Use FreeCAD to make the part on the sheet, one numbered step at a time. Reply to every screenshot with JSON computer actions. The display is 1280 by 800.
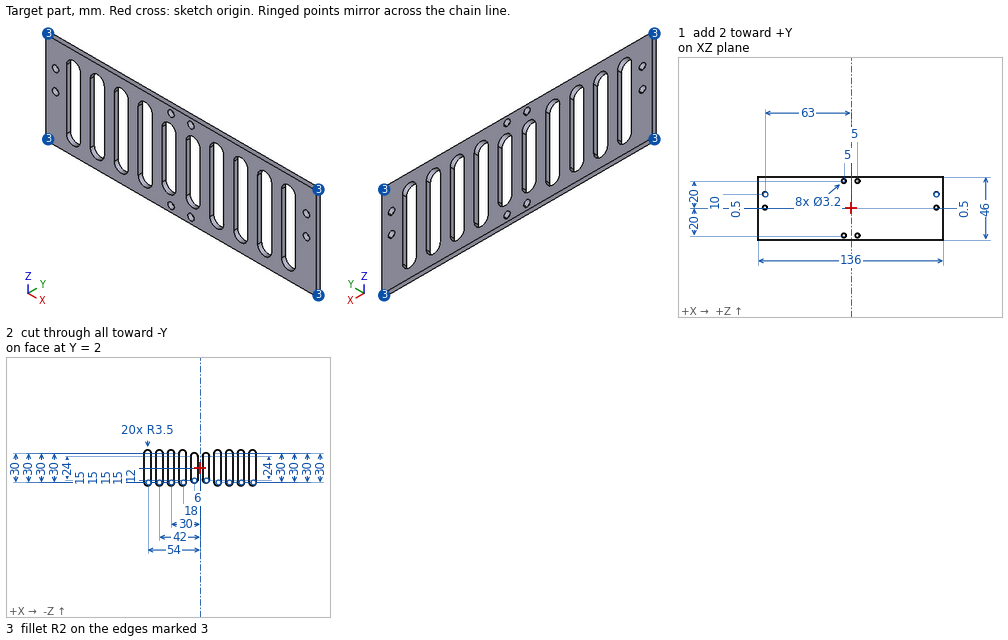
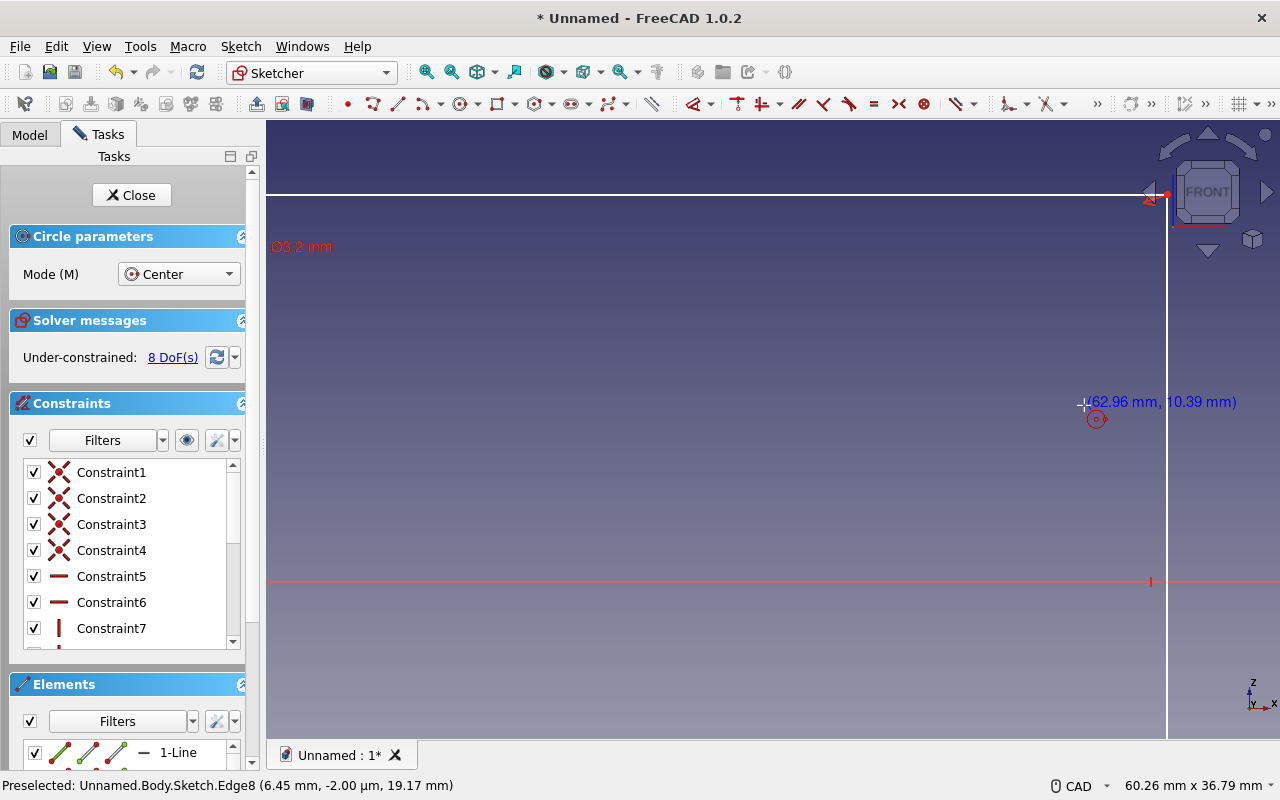
{"action": "scroll", "coordinate": [927, 380], "scroll_direction": "down", "scroll_amount": 7}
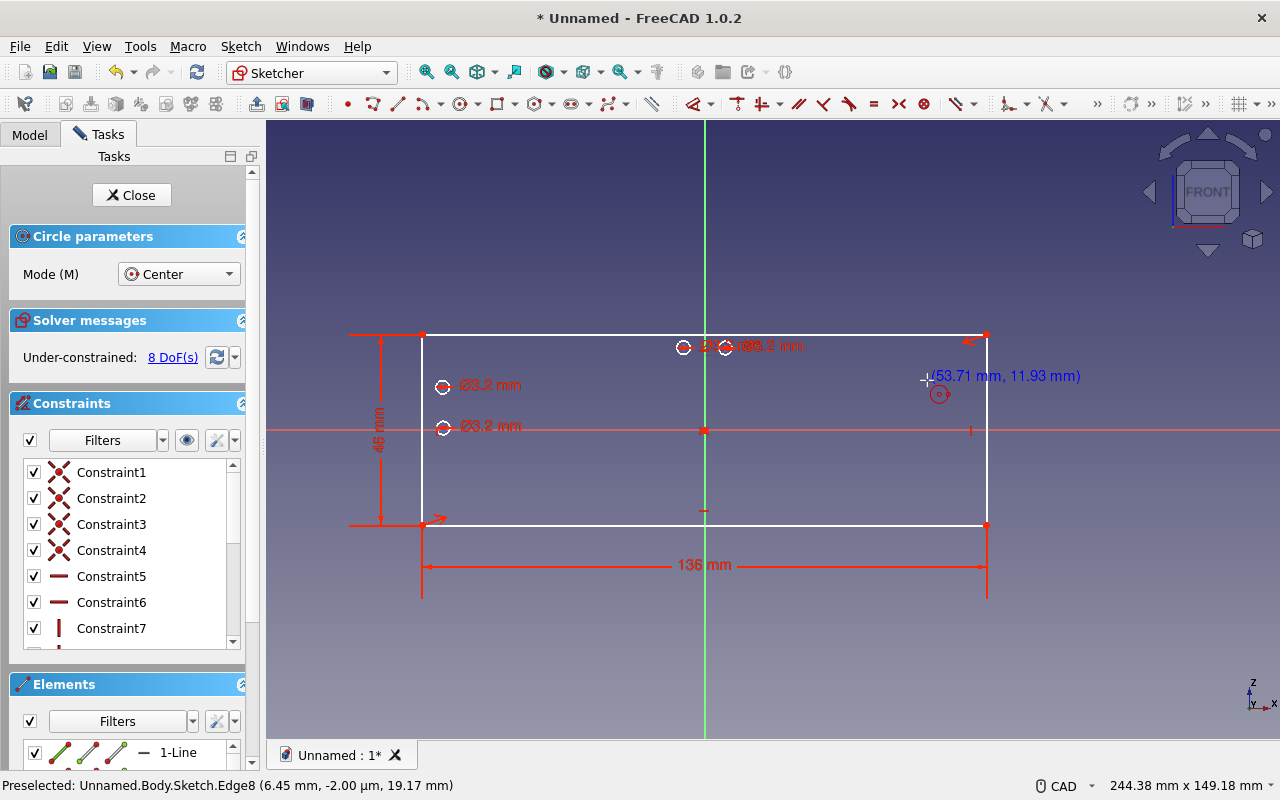
{"action": "left_click", "coordinate": [966, 387]}
{"action": "mouse_move", "coordinate": [971, 382]}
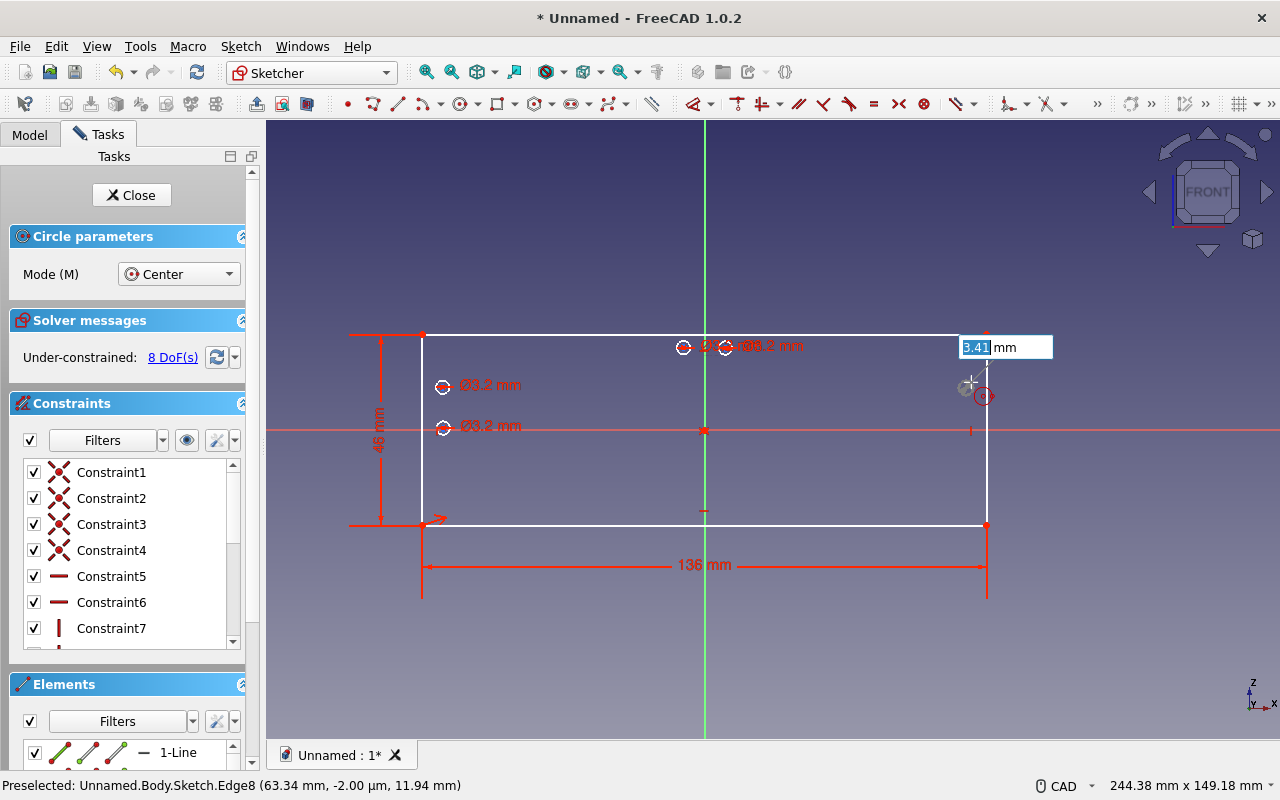
{"action": "type", "text": "3.2"}
{"action": "key", "text": "Return"}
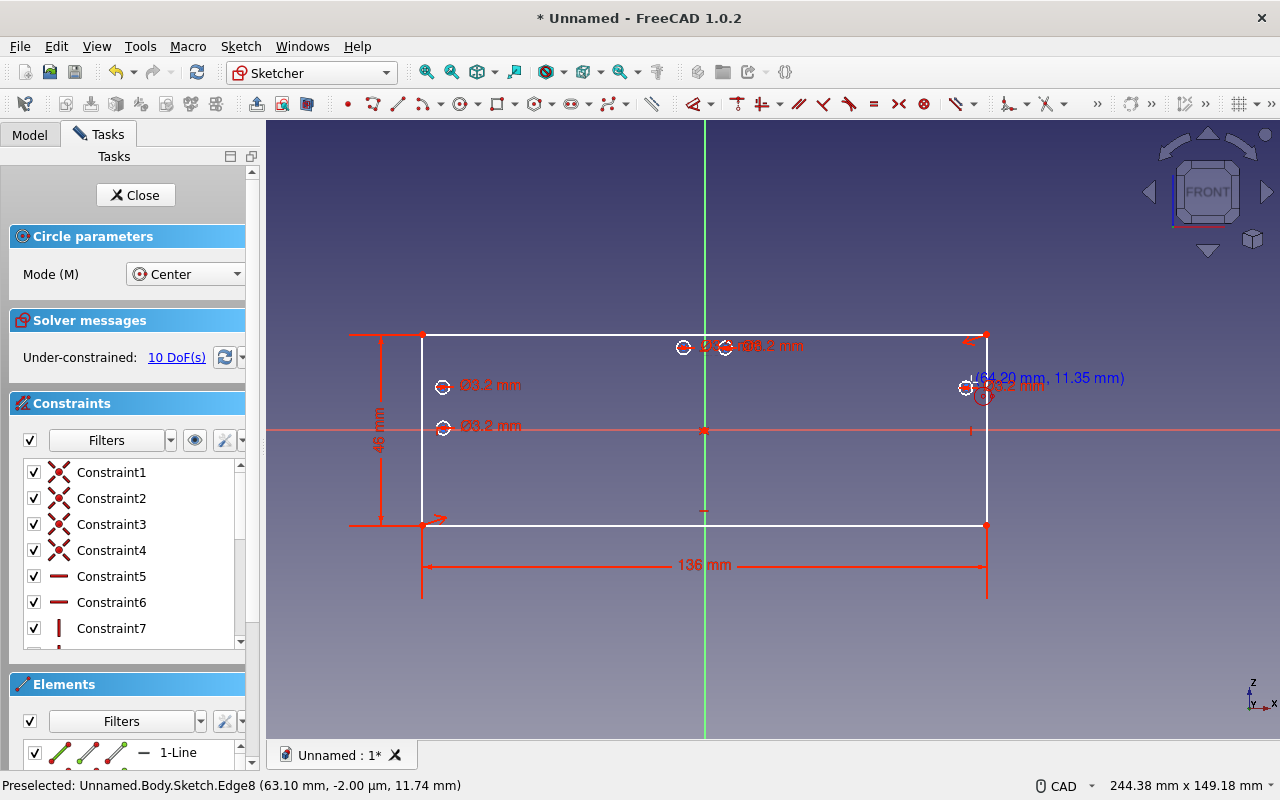
{"action": "scroll", "coordinate": [966, 428], "scroll_direction": "up", "scroll_amount": 11}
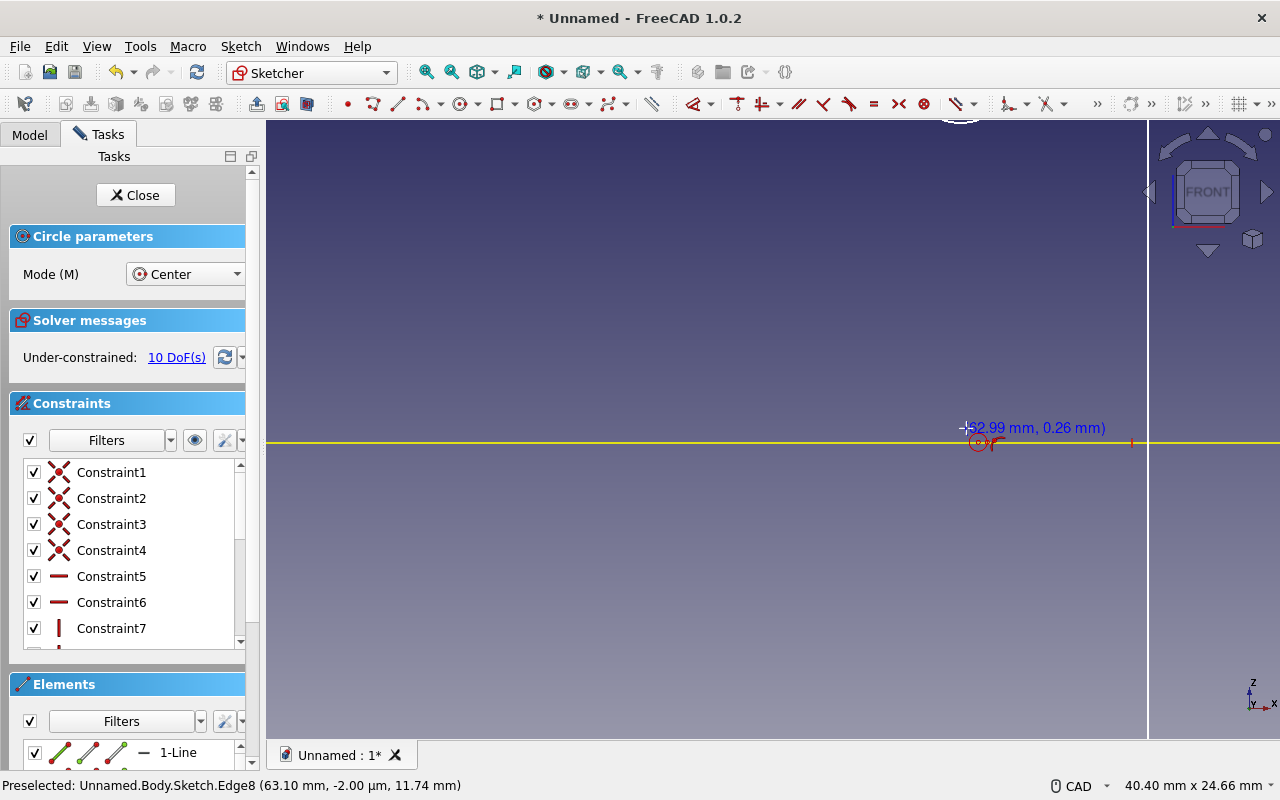
{"action": "left_click", "coordinate": [961, 424]}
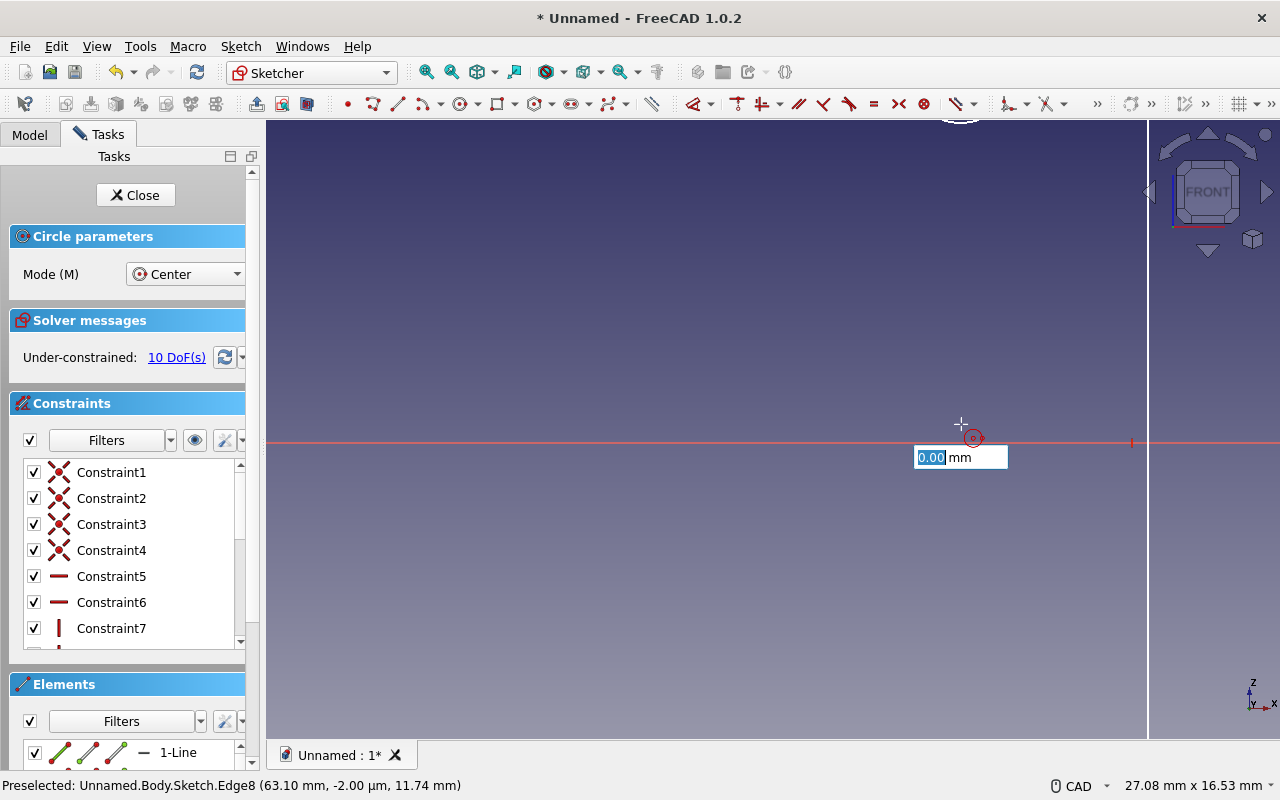
{"action": "scroll", "coordinate": [967, 428], "scroll_direction": "down", "scroll_amount": 11}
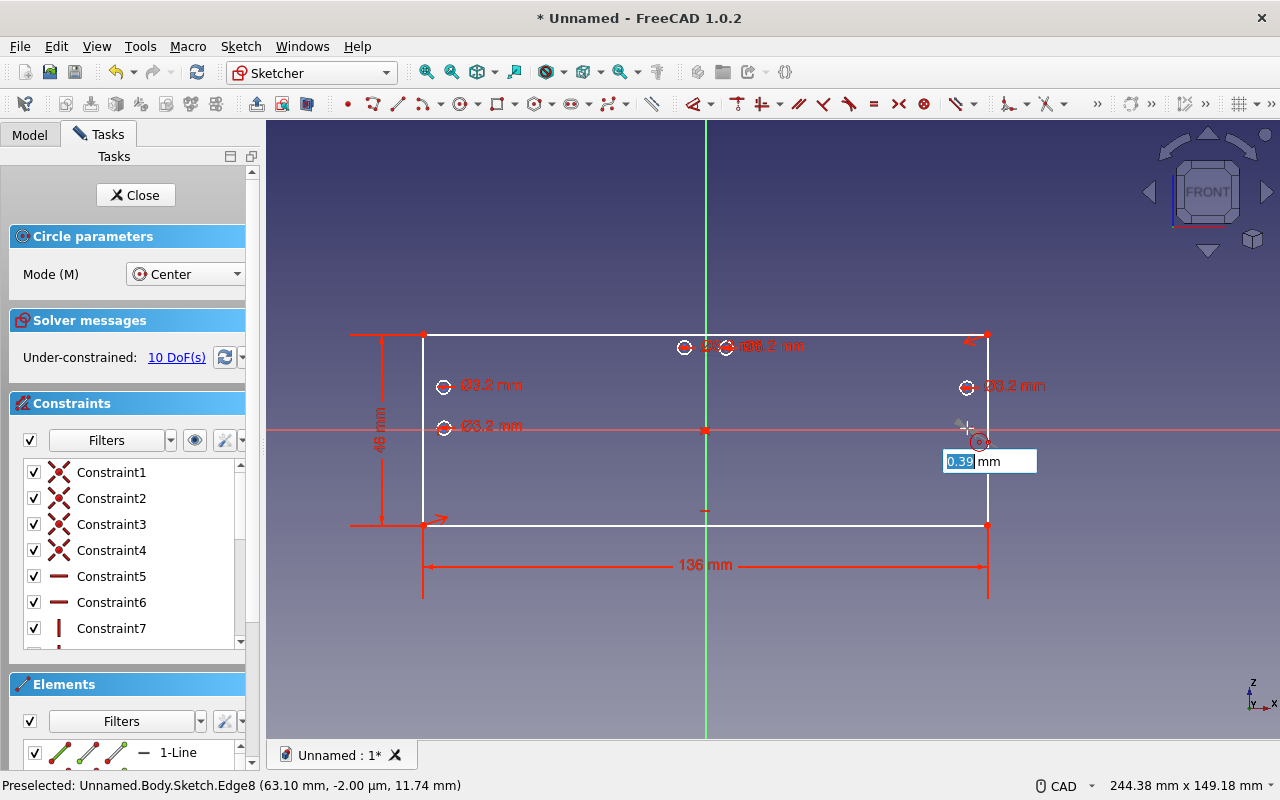
{"action": "scroll", "coordinate": [972, 423], "scroll_direction": "up", "scroll_amount": 5}
{"action": "mouse_move", "coordinate": [970, 423]}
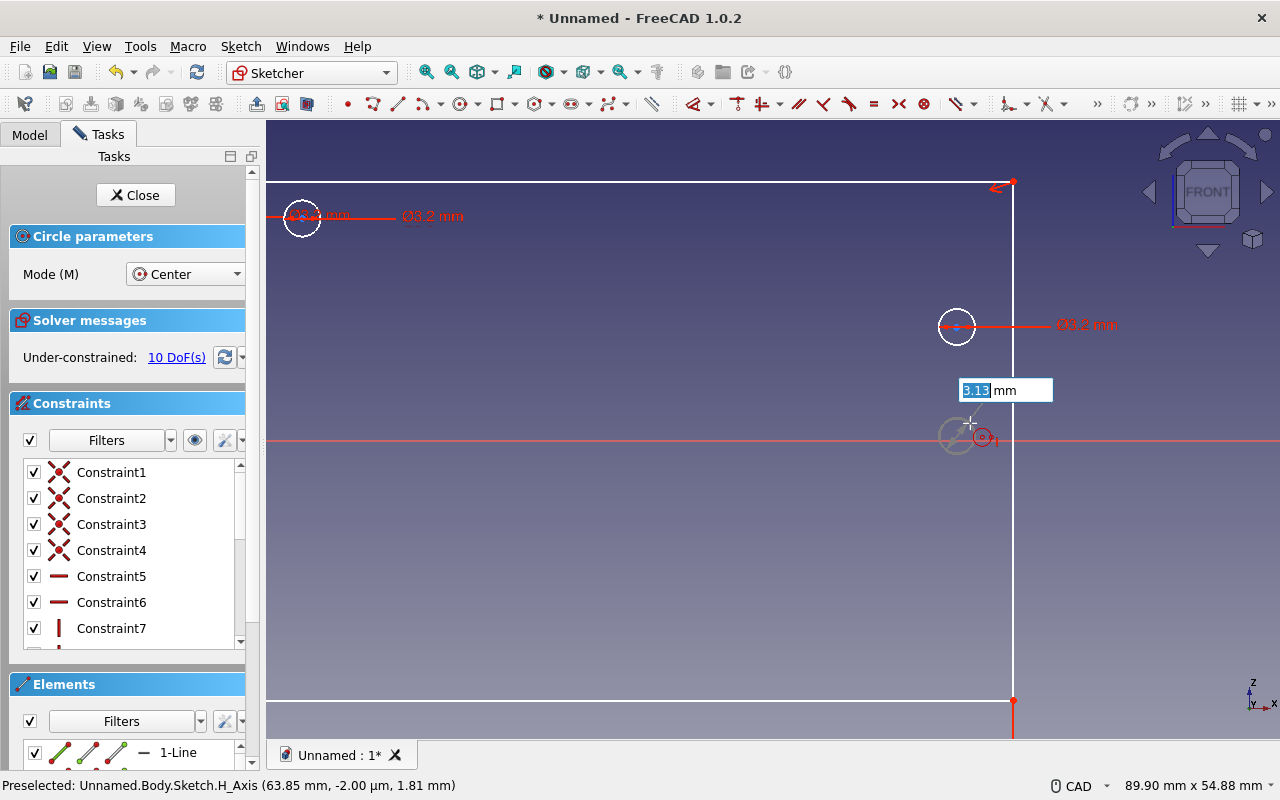
{"action": "type", "text": "3.2"}
{"action": "key", "text": "Return"}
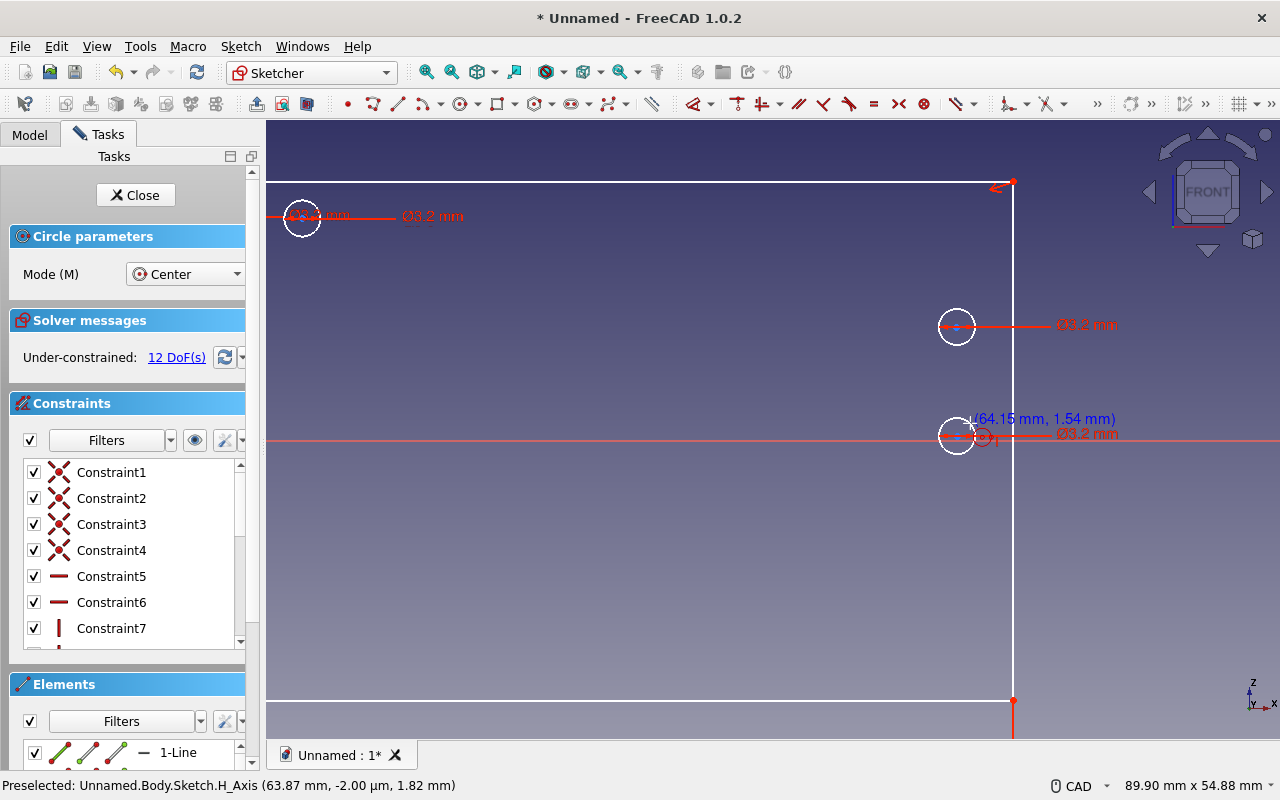
{"action": "scroll", "coordinate": [971, 423], "scroll_direction": "down", "scroll_amount": 5}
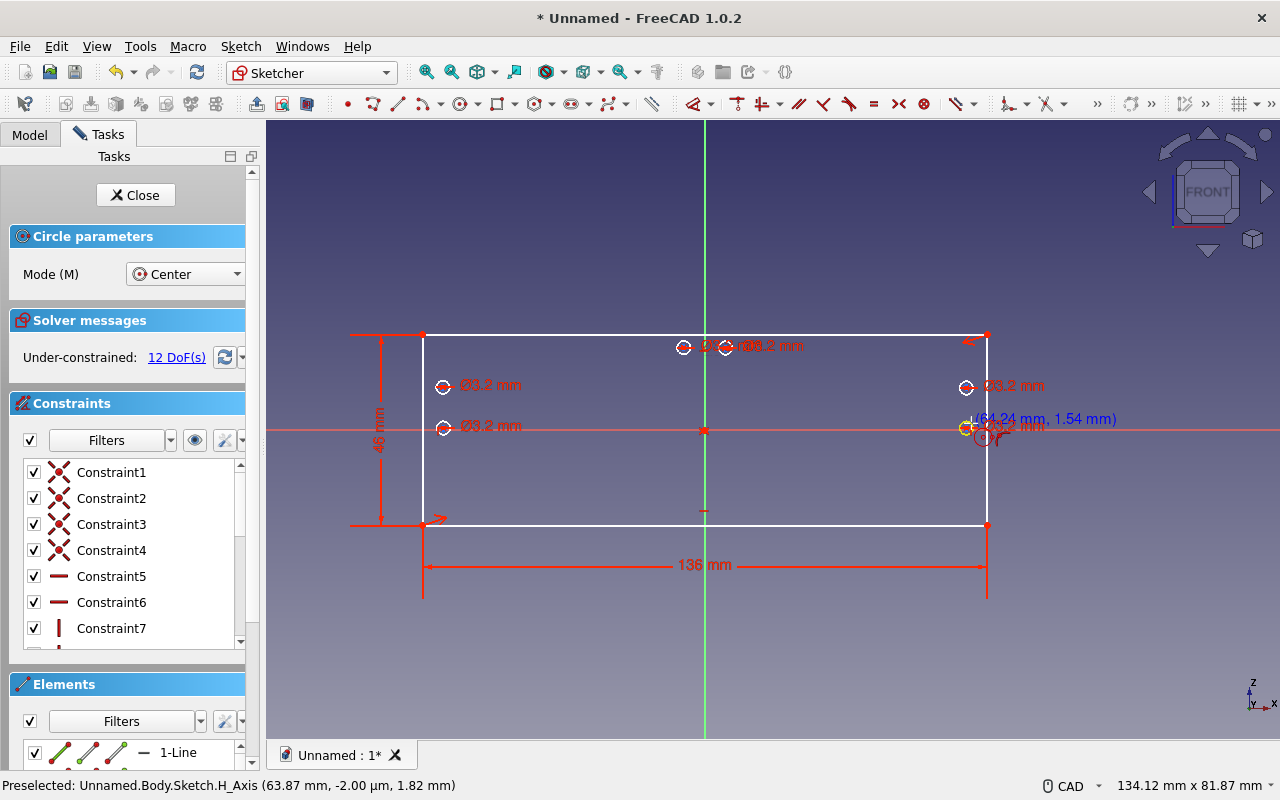
{"action": "scroll", "coordinate": [684, 513], "scroll_direction": "up", "scroll_amount": 7}